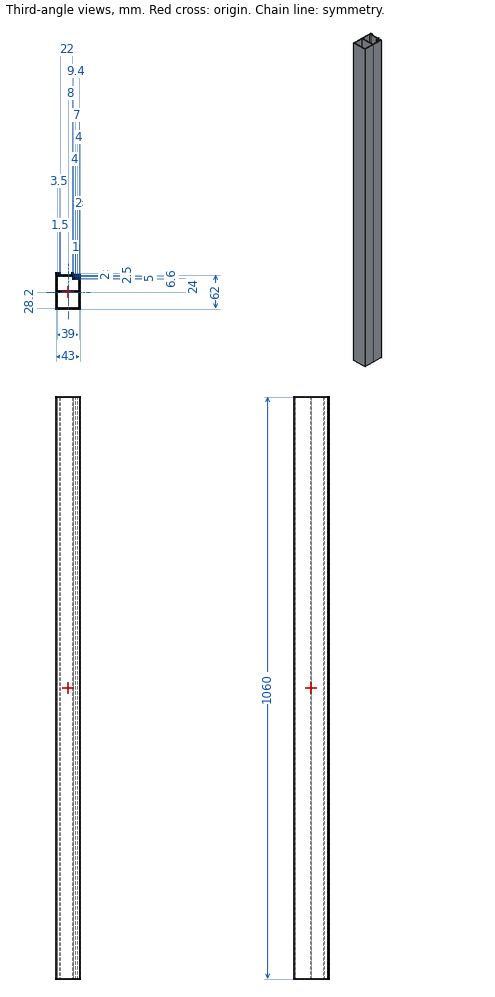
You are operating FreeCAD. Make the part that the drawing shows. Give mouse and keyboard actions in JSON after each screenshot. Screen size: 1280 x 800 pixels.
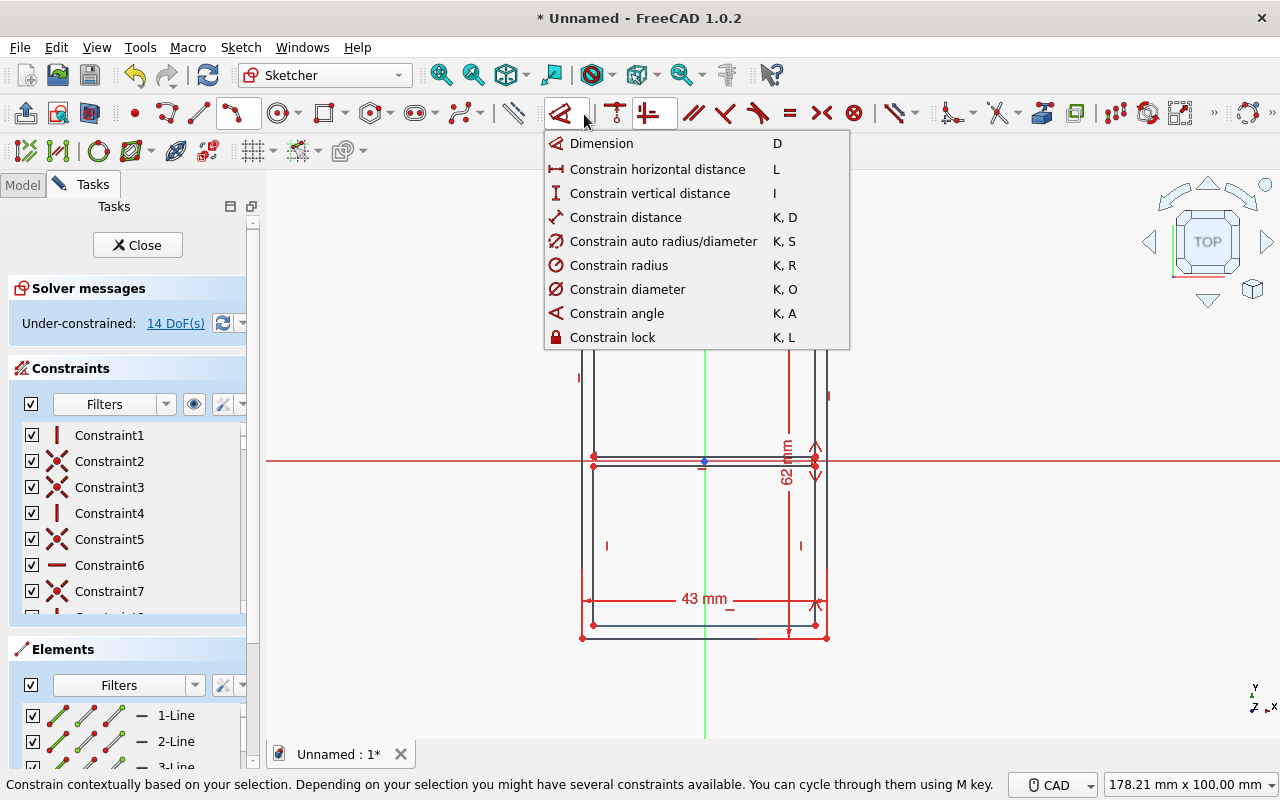
{"action": "left_click", "coordinate": [697, 169]}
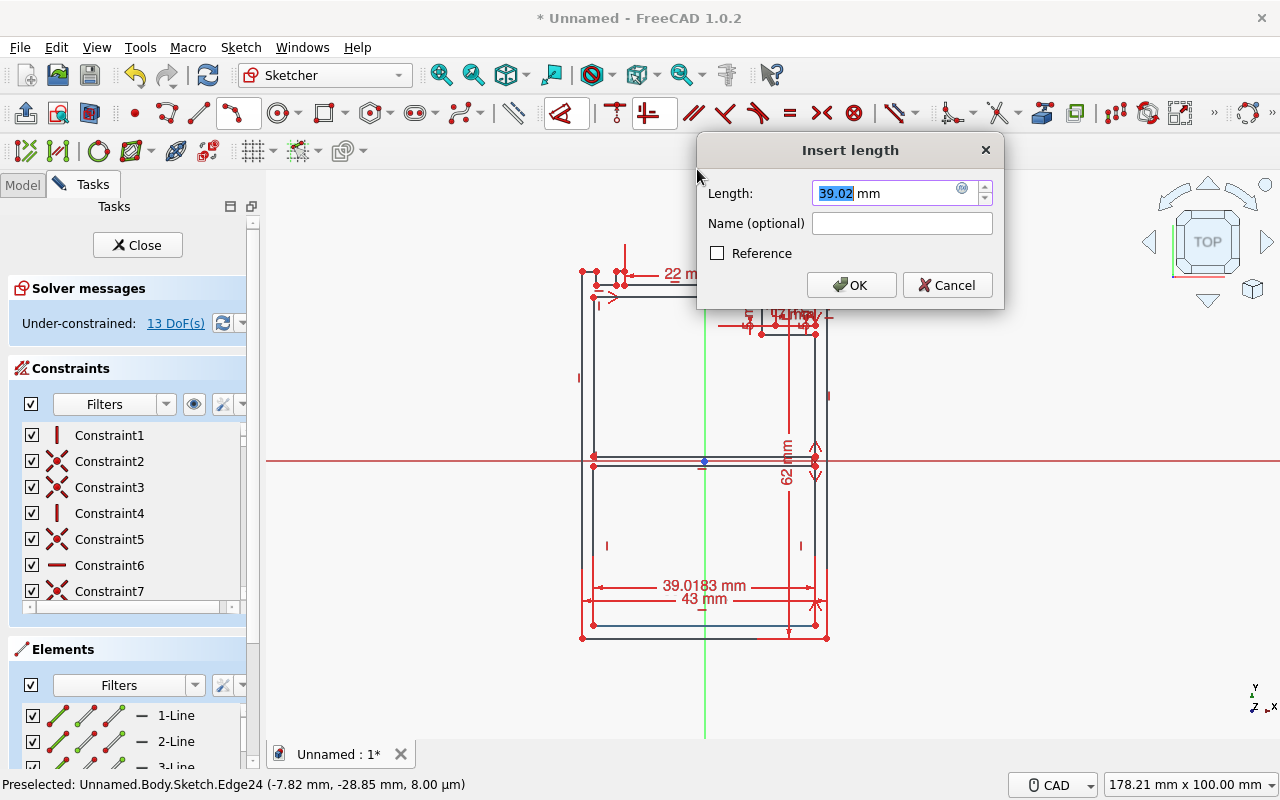
{"action": "type", "text": "39"}
{"action": "key", "text": "Return"}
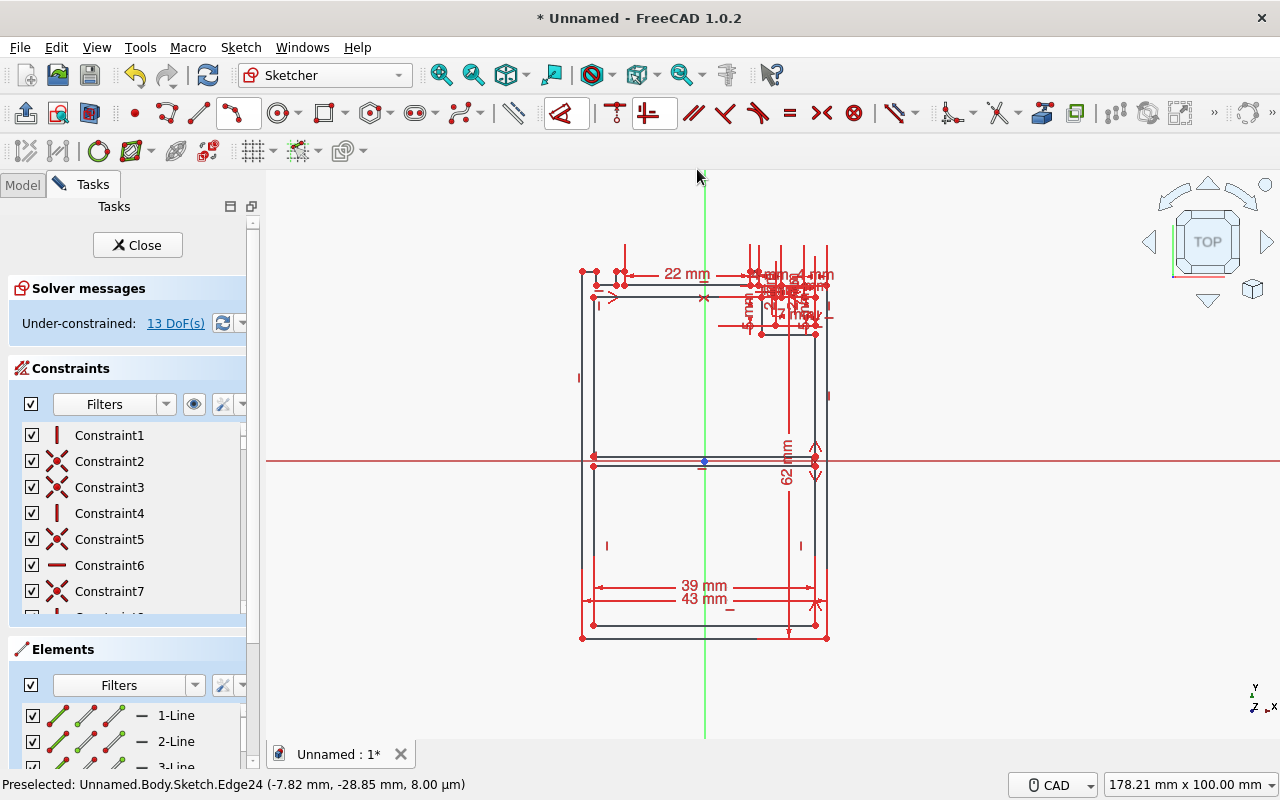
{"action": "scroll", "coordinate": [749, 457], "scroll_direction": "up", "scroll_amount": 6}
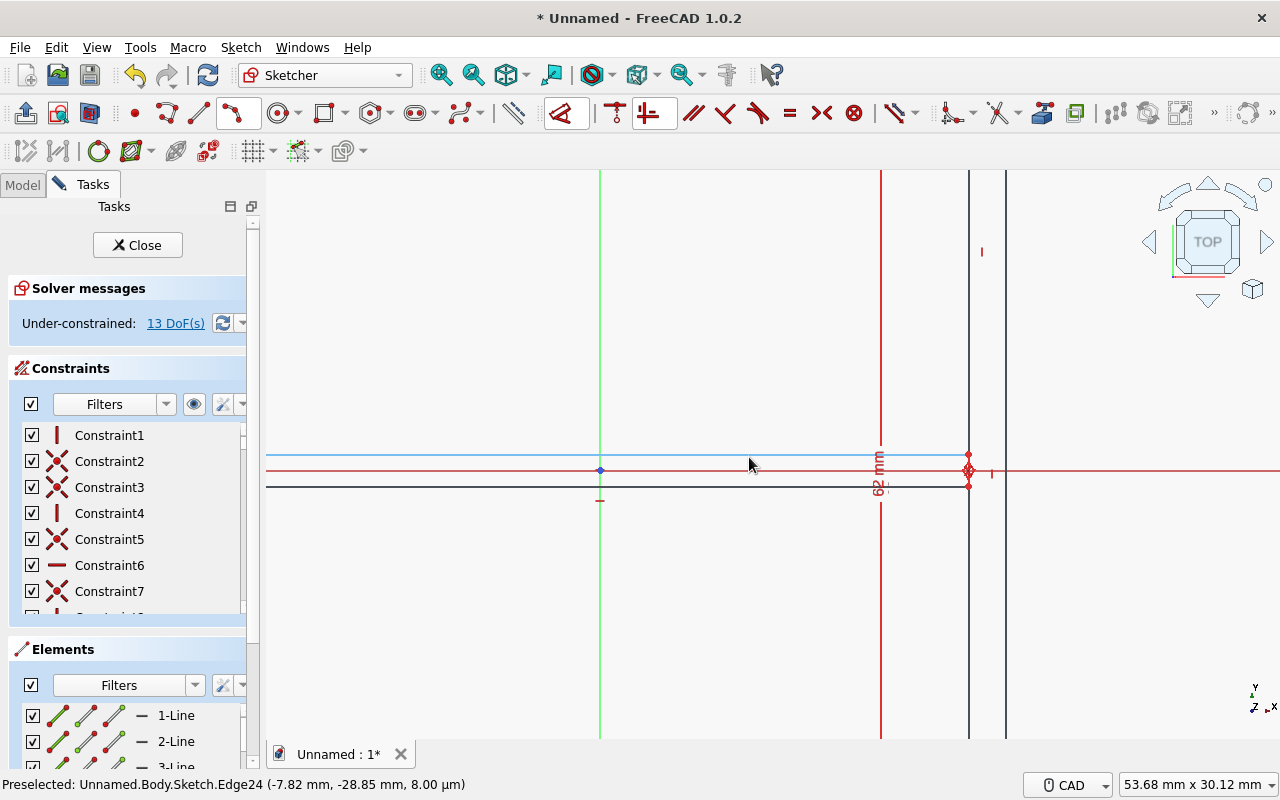
{"action": "left_click", "coordinate": [748, 455]}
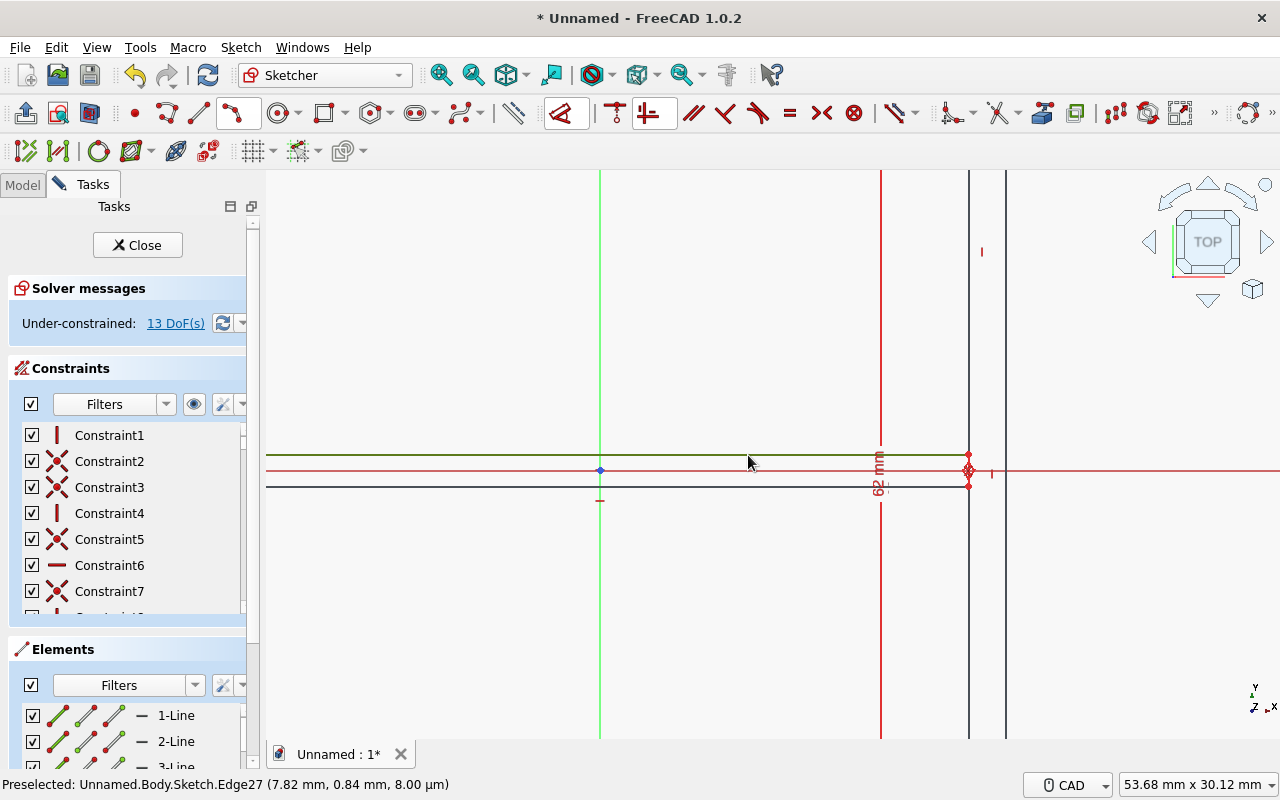
{"action": "left_click", "coordinate": [584, 114]}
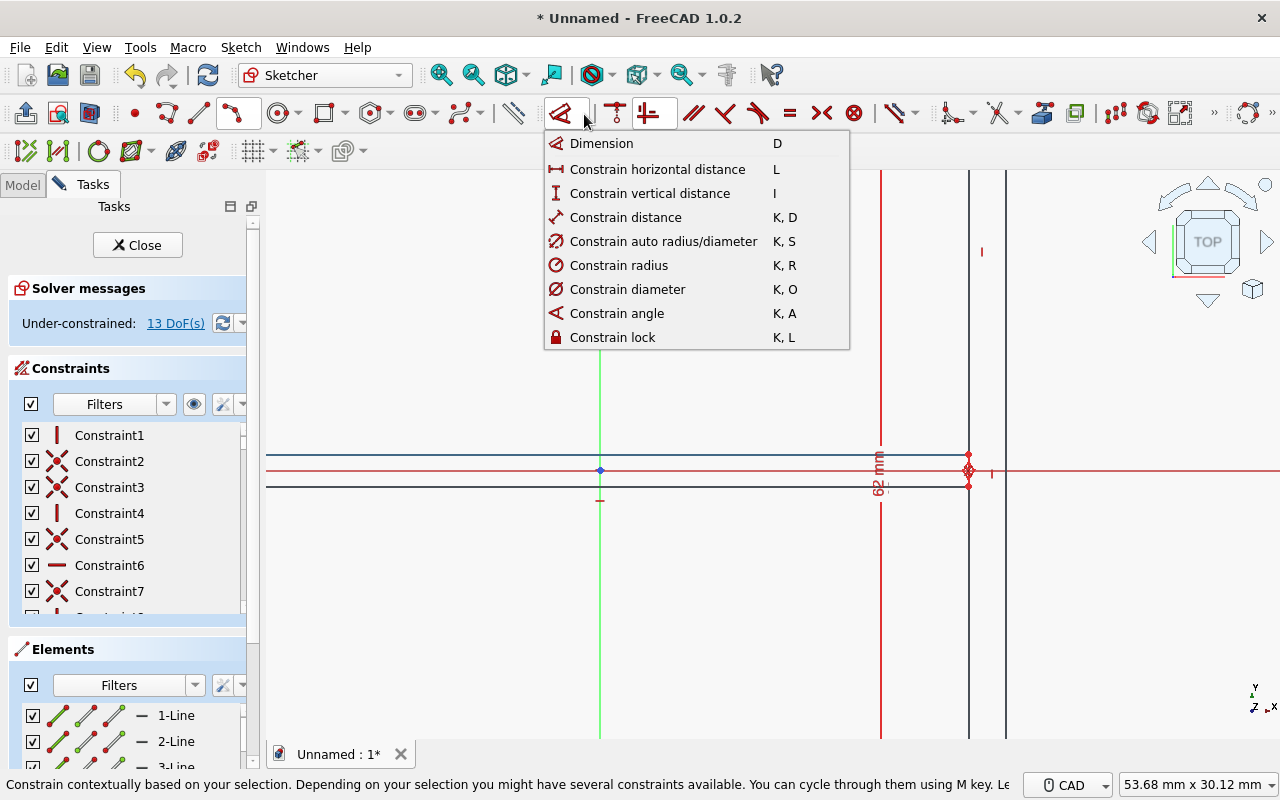
{"action": "left_click", "coordinate": [697, 169]}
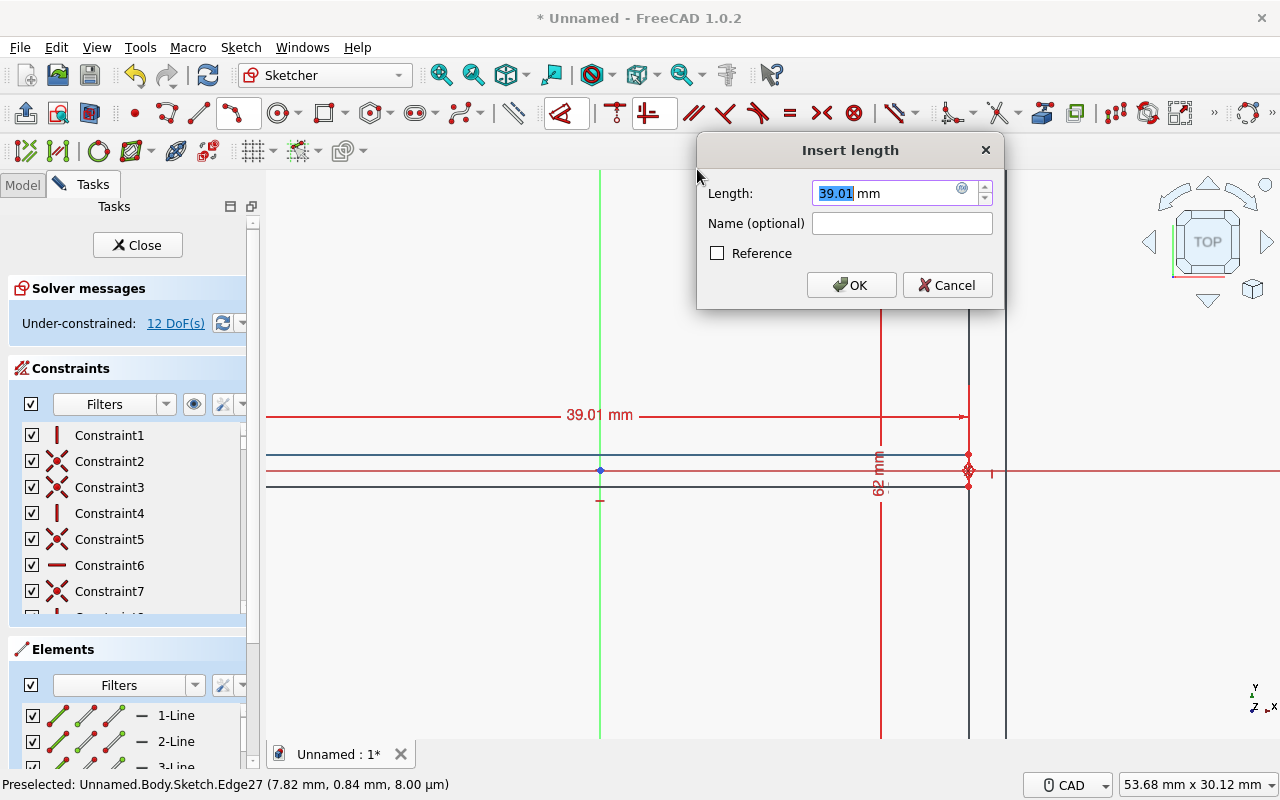
{"action": "type", "text": "39"}
{"action": "key", "text": "Return"}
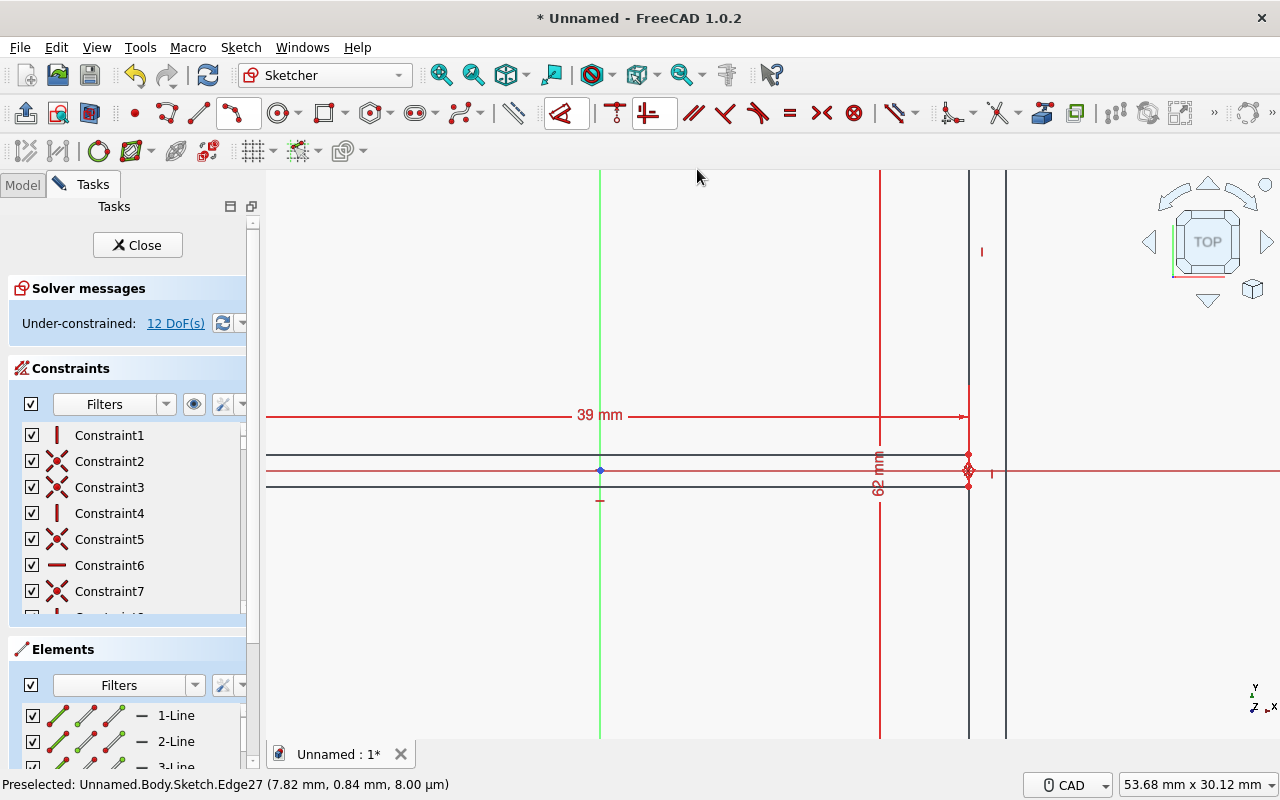
{"action": "scroll", "coordinate": [749, 458], "scroll_direction": "down", "scroll_amount": 6}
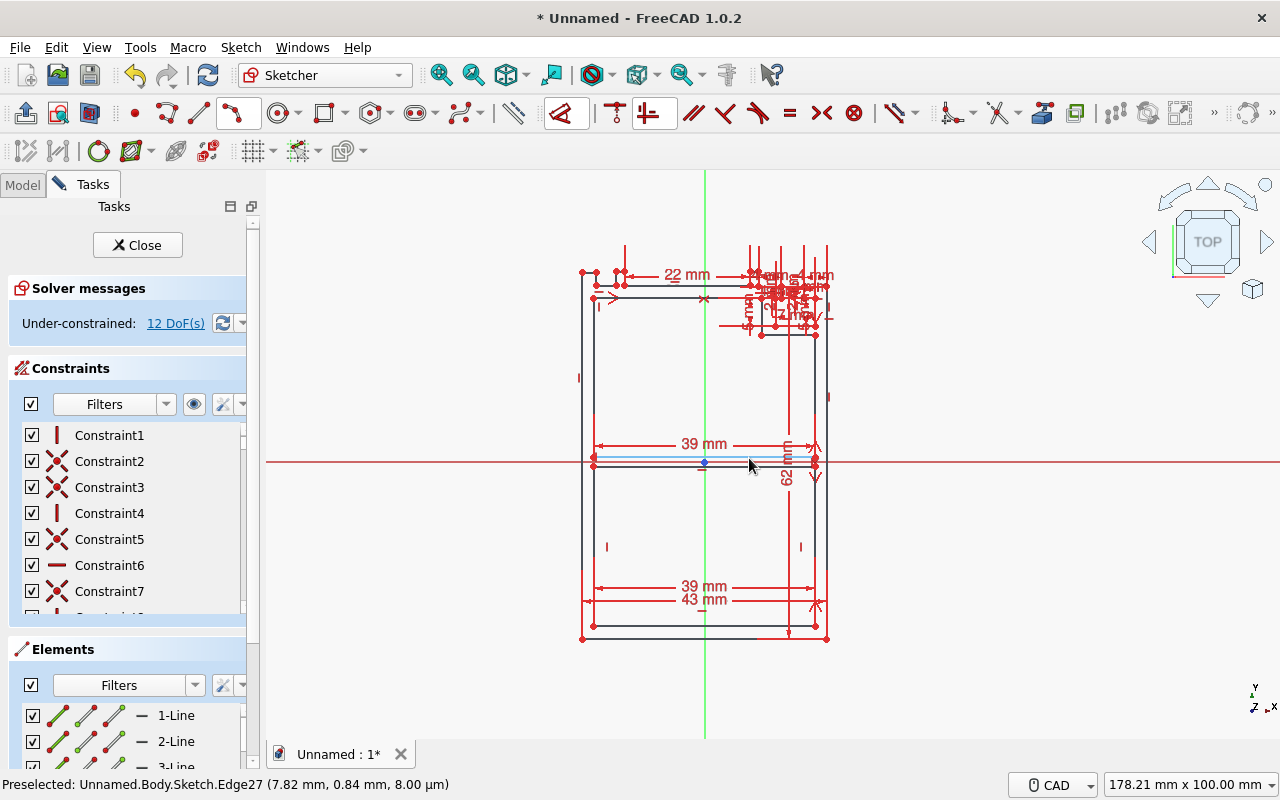
{"action": "scroll", "coordinate": [750, 272], "scroll_direction": "up", "scroll_amount": 2}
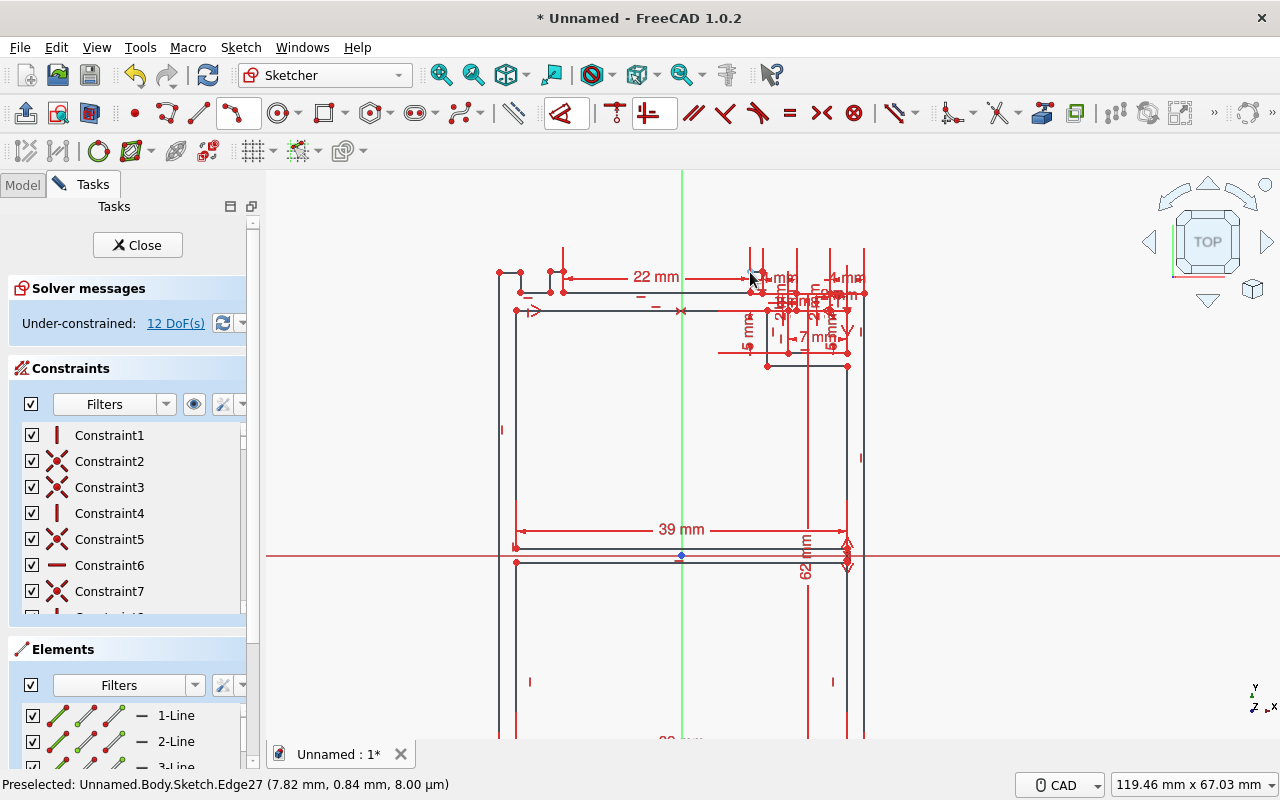
{"action": "left_click", "coordinate": [750, 272]}